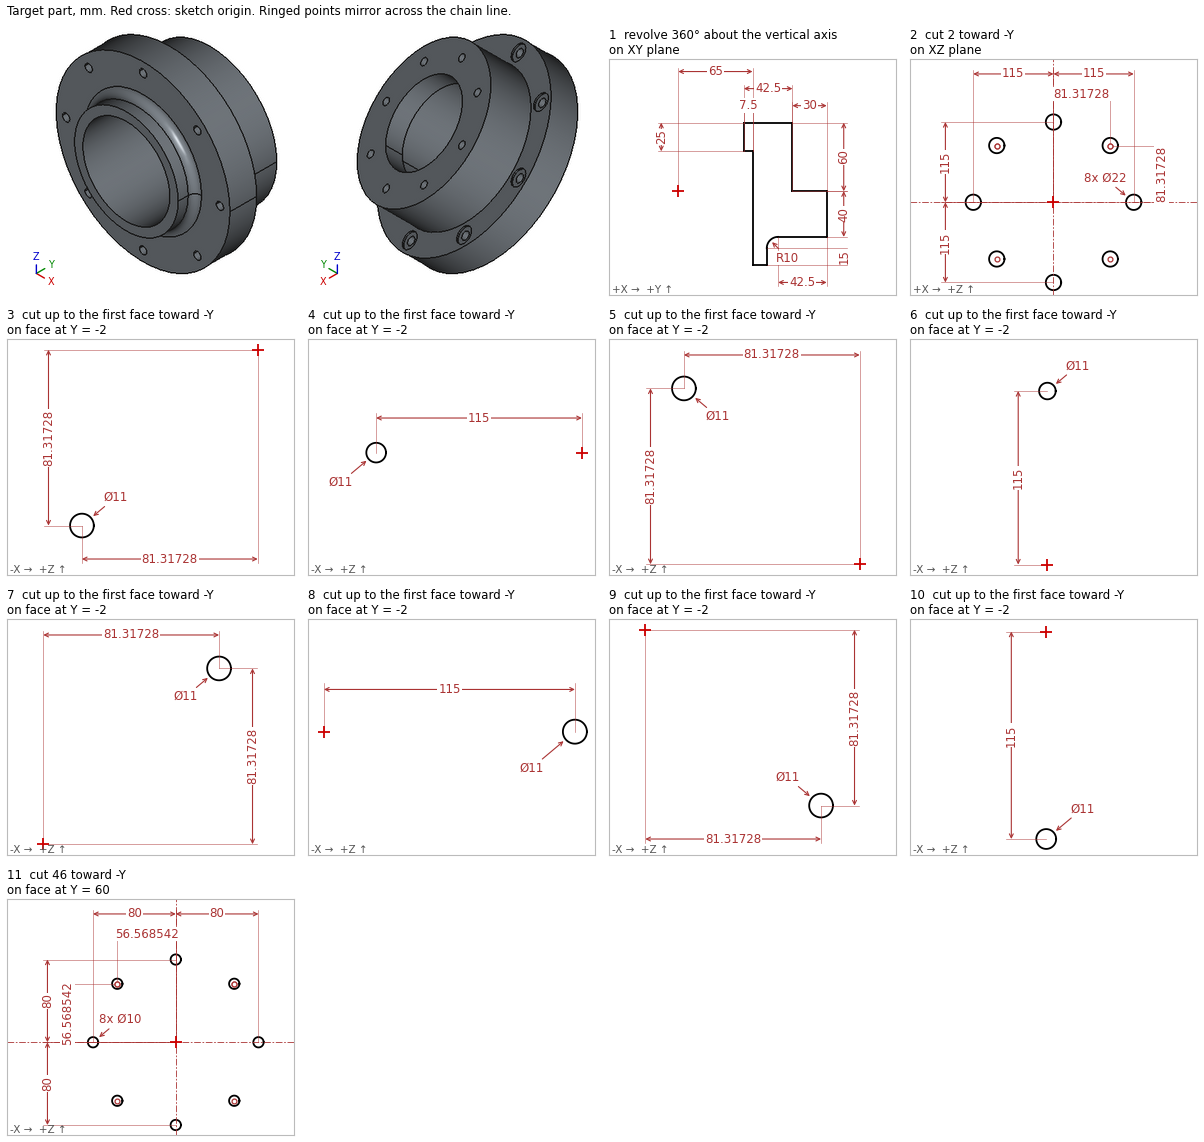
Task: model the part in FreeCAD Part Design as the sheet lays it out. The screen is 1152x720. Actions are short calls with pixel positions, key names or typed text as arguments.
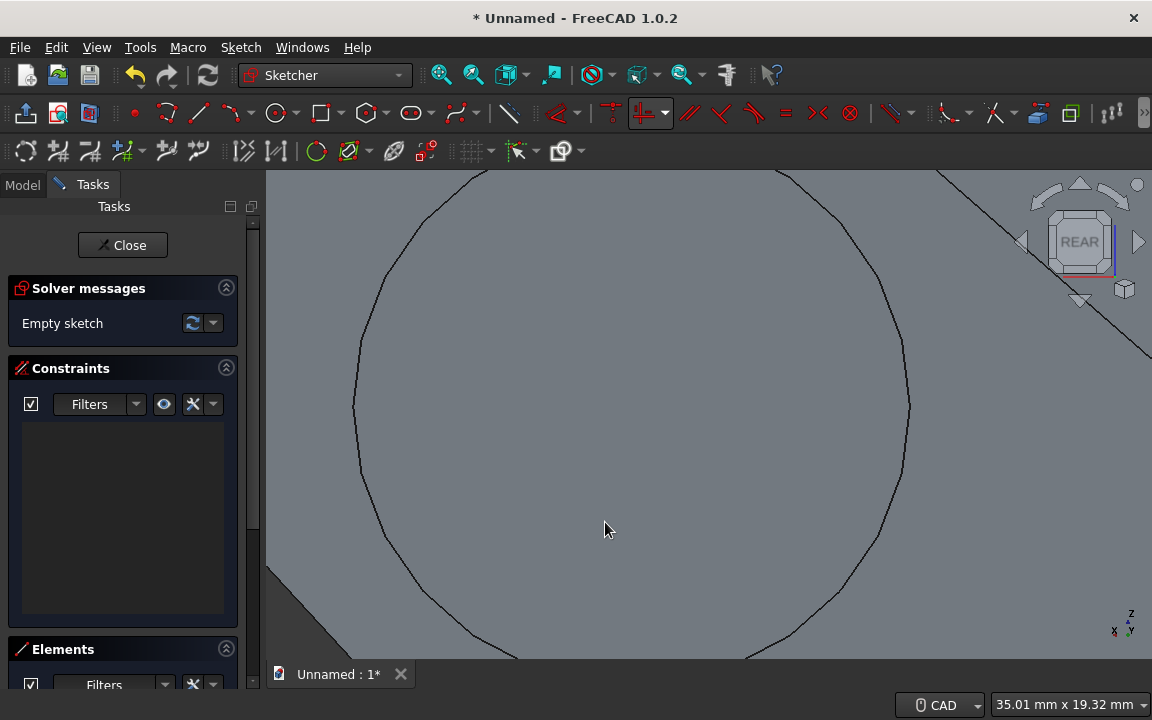
click(276, 114)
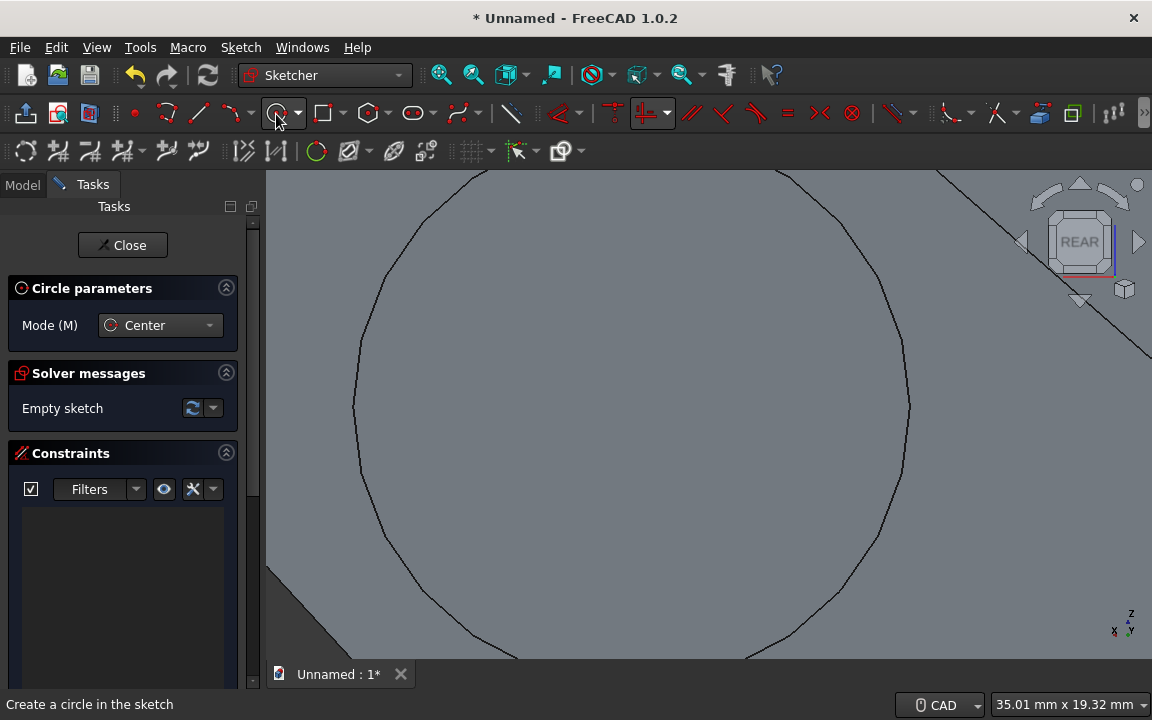
click(632, 407)
move(730, 308)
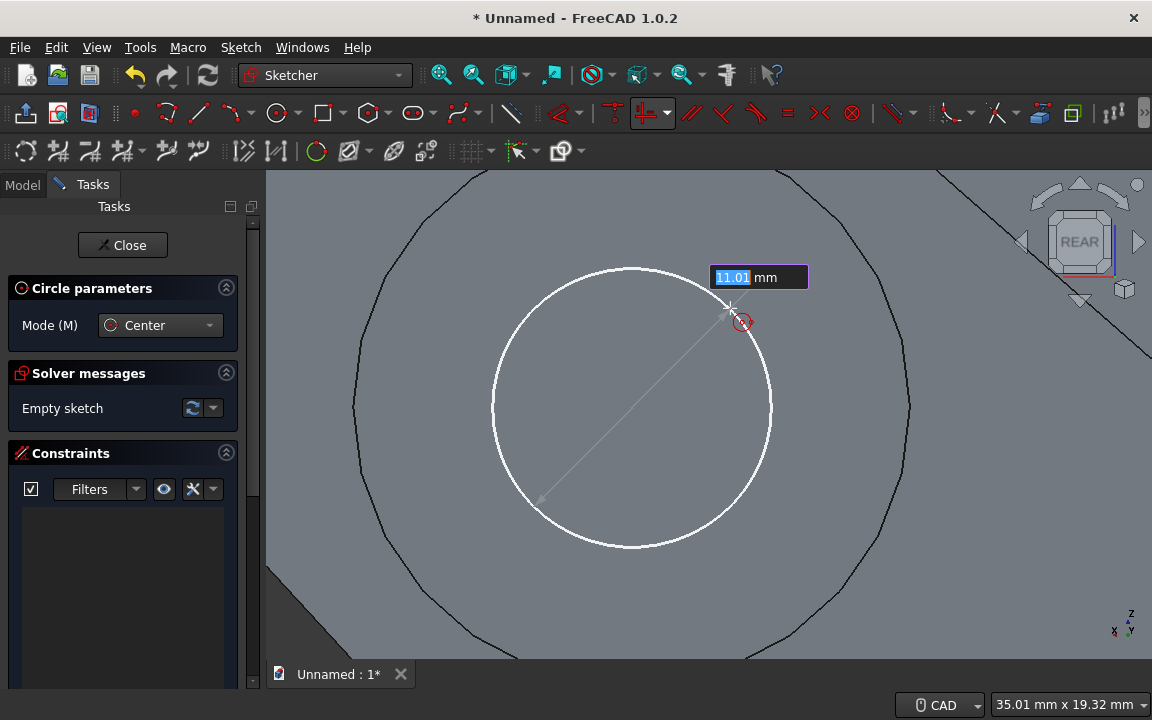
text(11)
key(Return)
key(Escape)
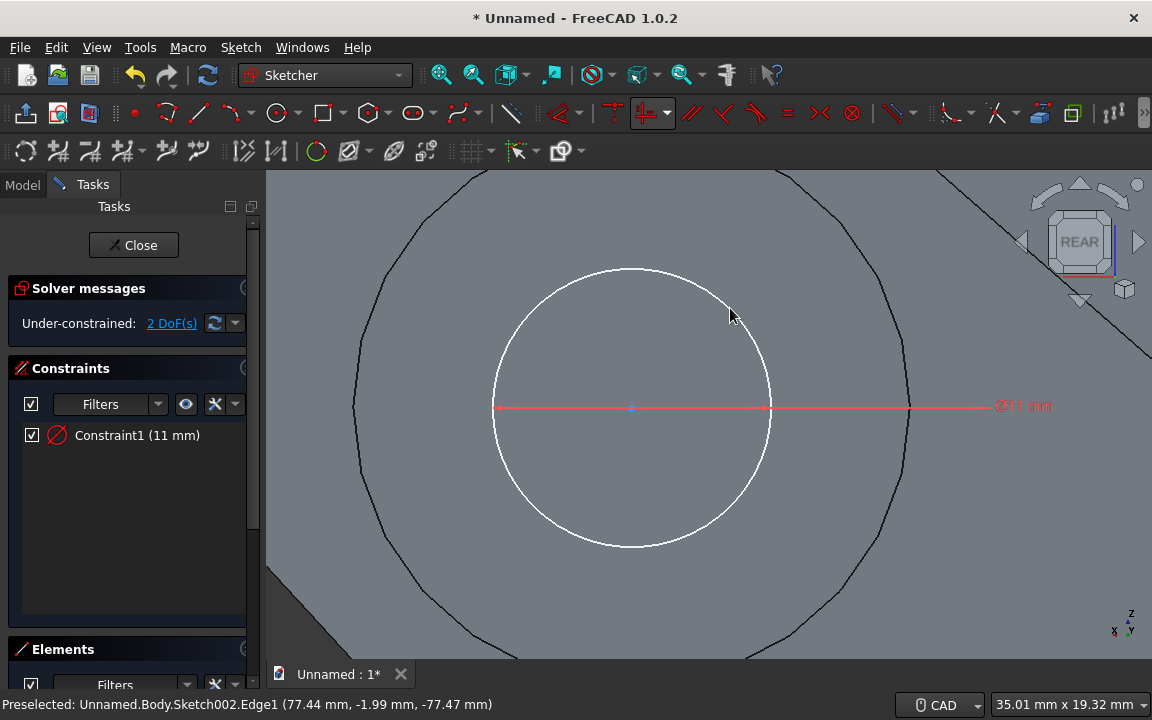
key(d)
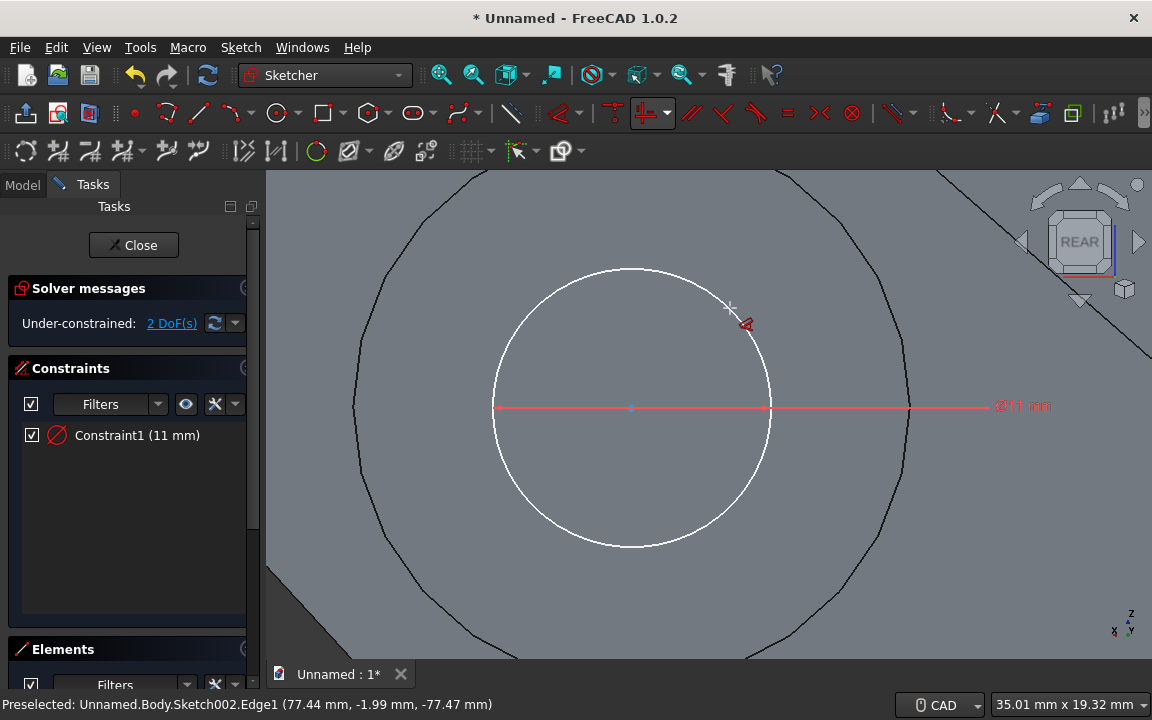
click(632, 408)
click(809, 442)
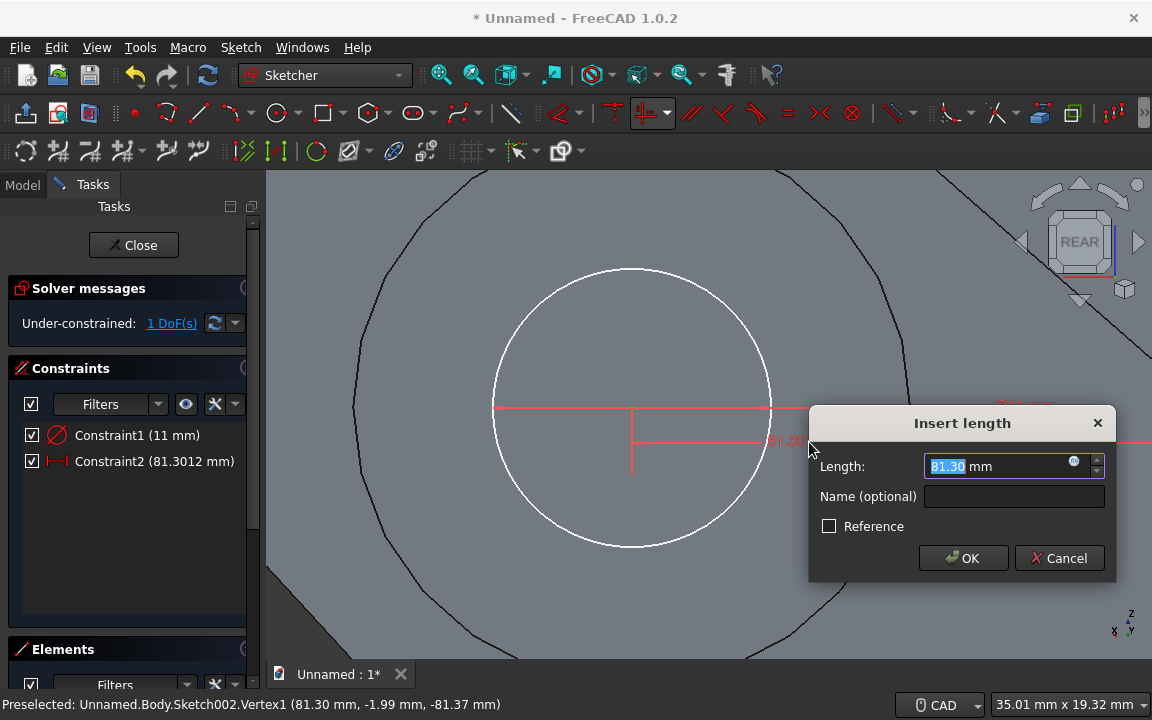
text(81.31728)
key(Return)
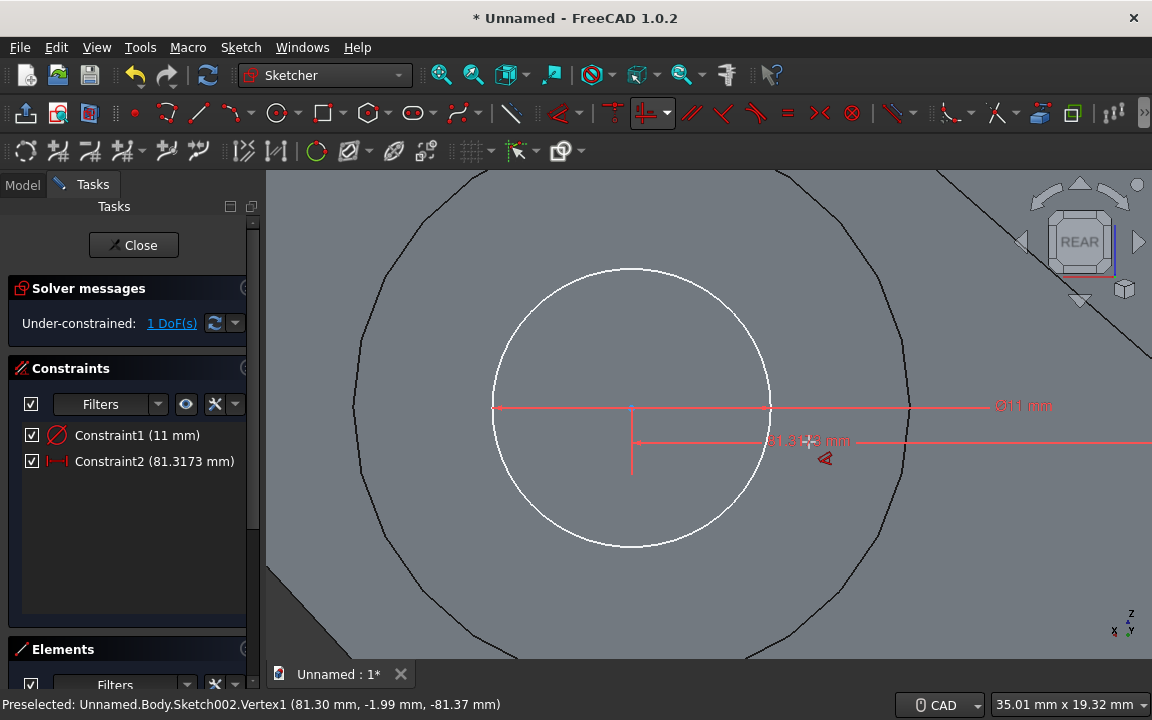
click(632, 408)
click(598, 303)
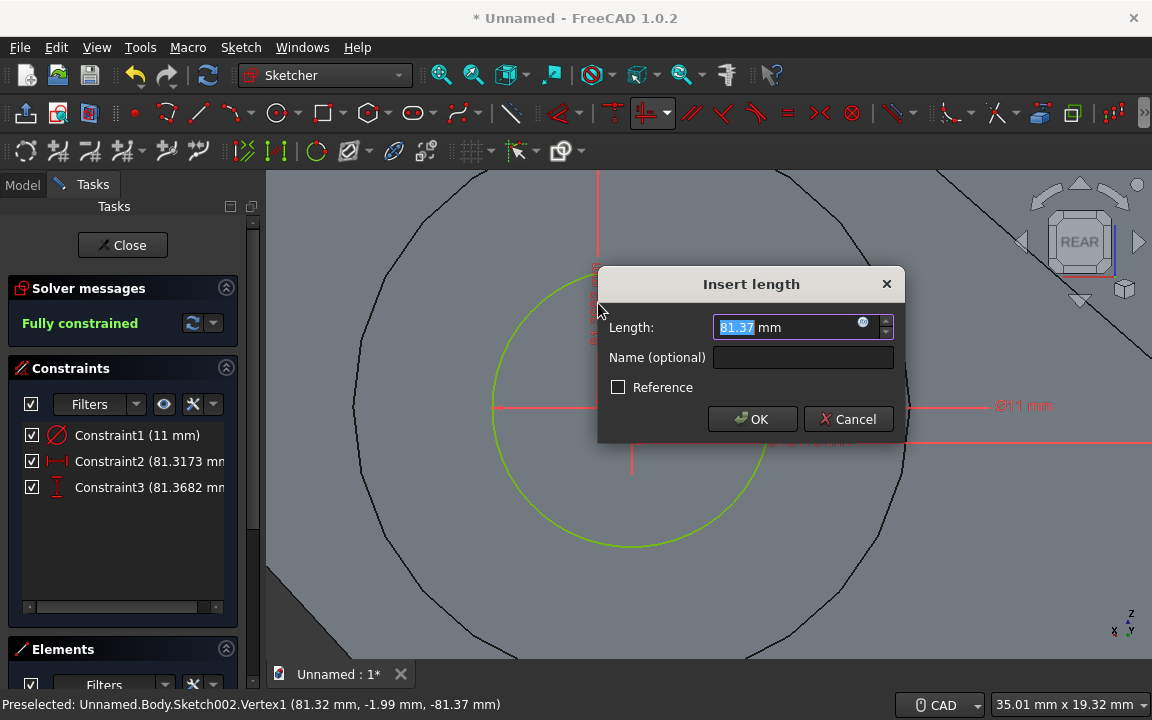
text(81.31728)
key(Return)
key(Escape)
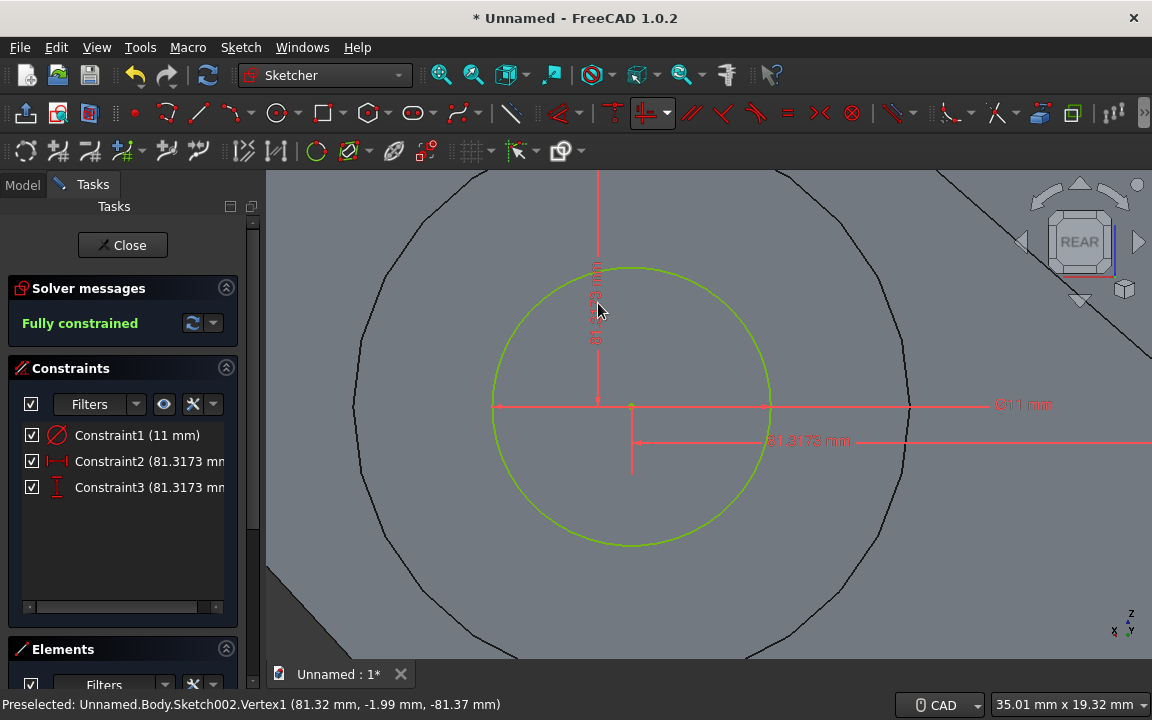
click(123, 245)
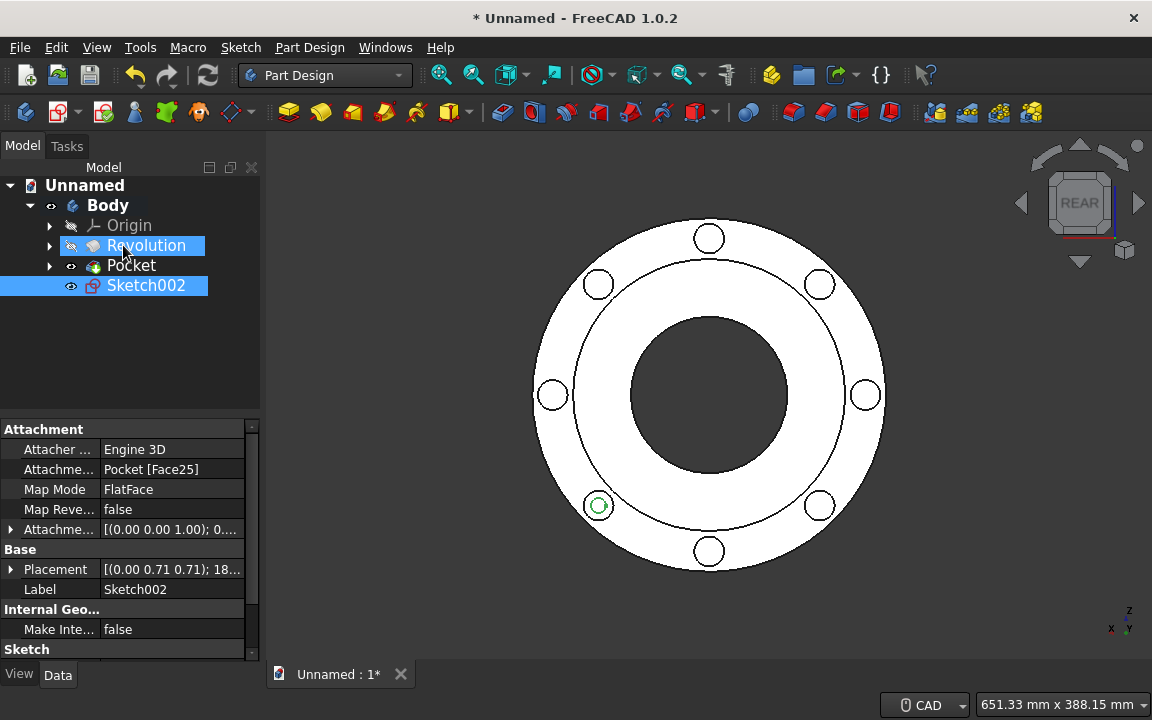
click(504, 112)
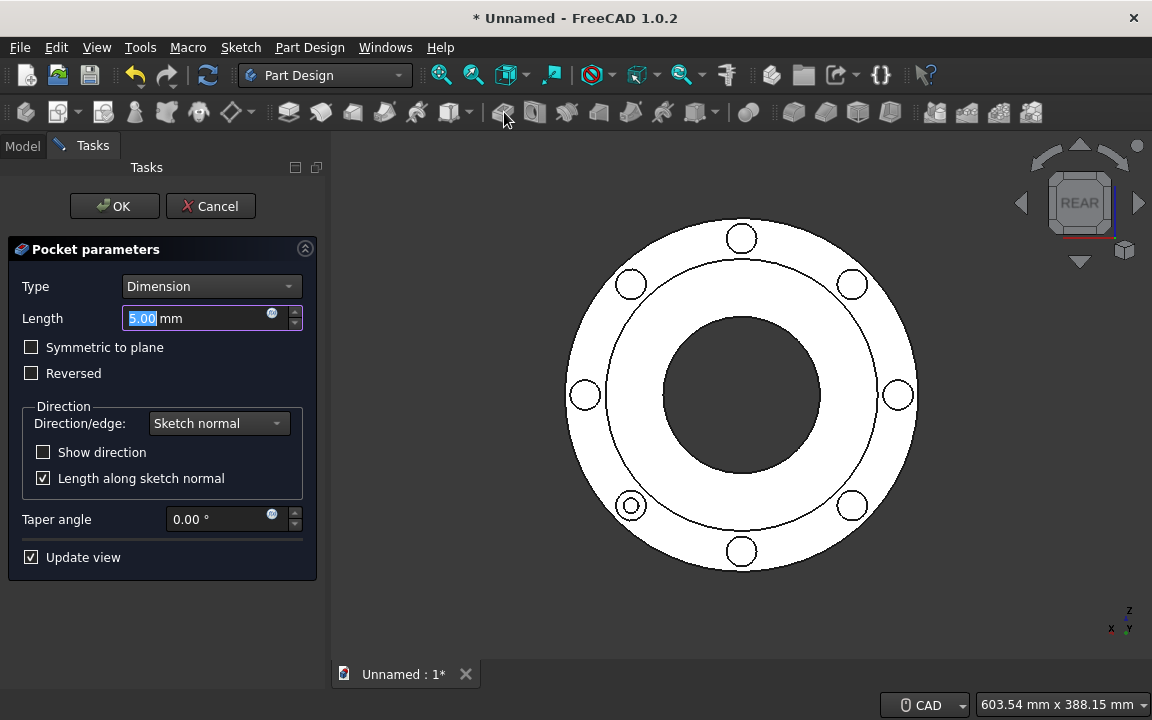
click(212, 286)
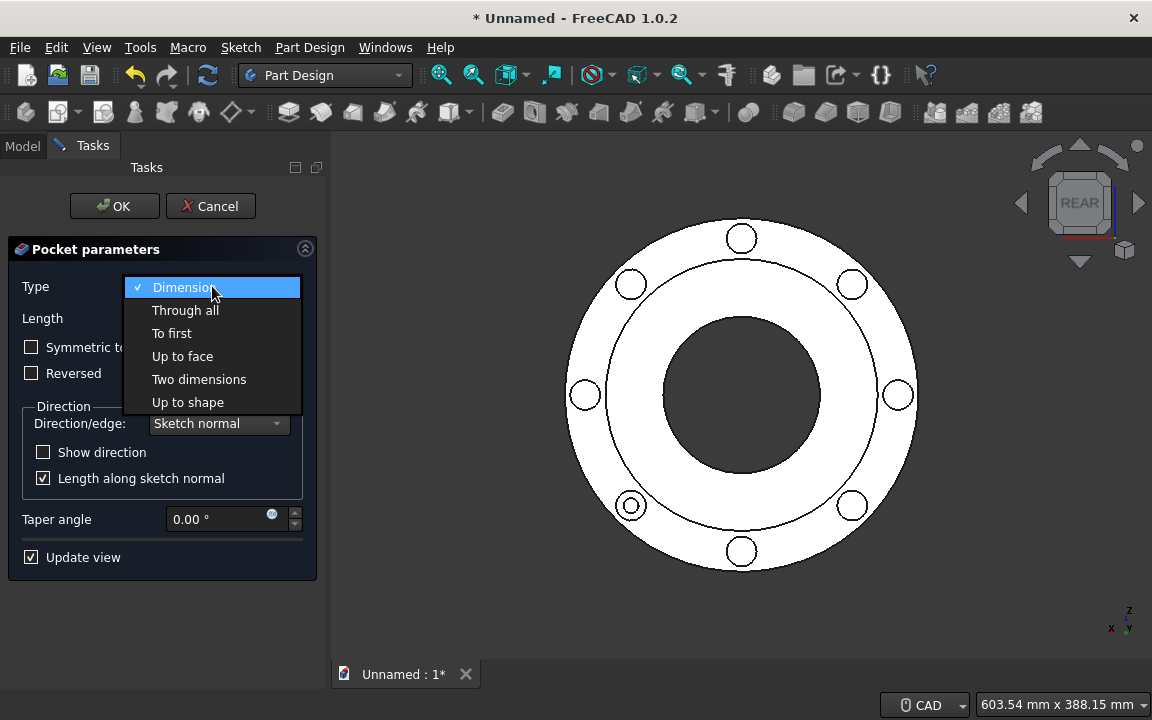
click(212, 334)